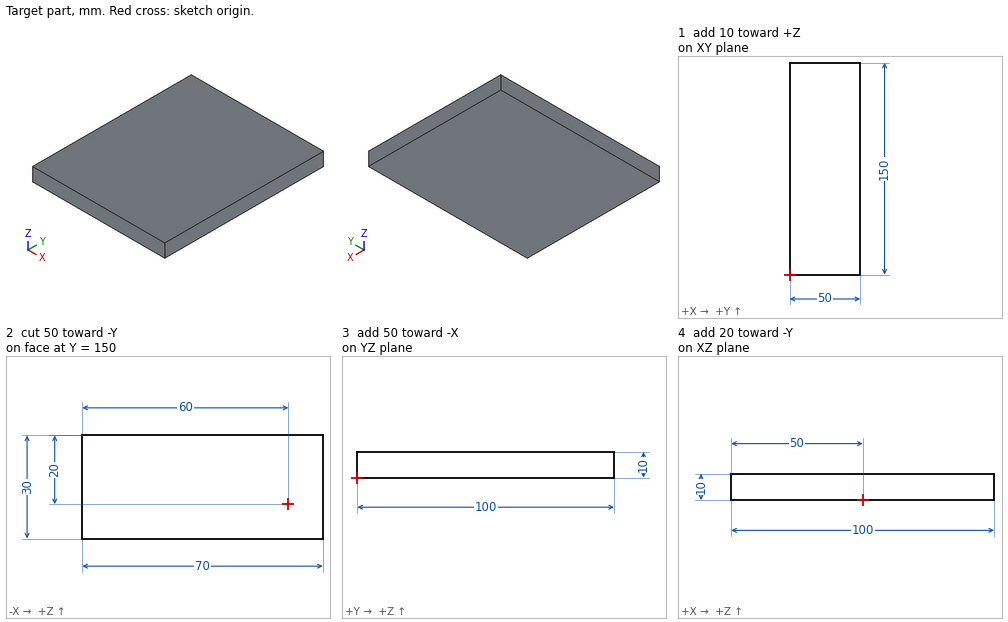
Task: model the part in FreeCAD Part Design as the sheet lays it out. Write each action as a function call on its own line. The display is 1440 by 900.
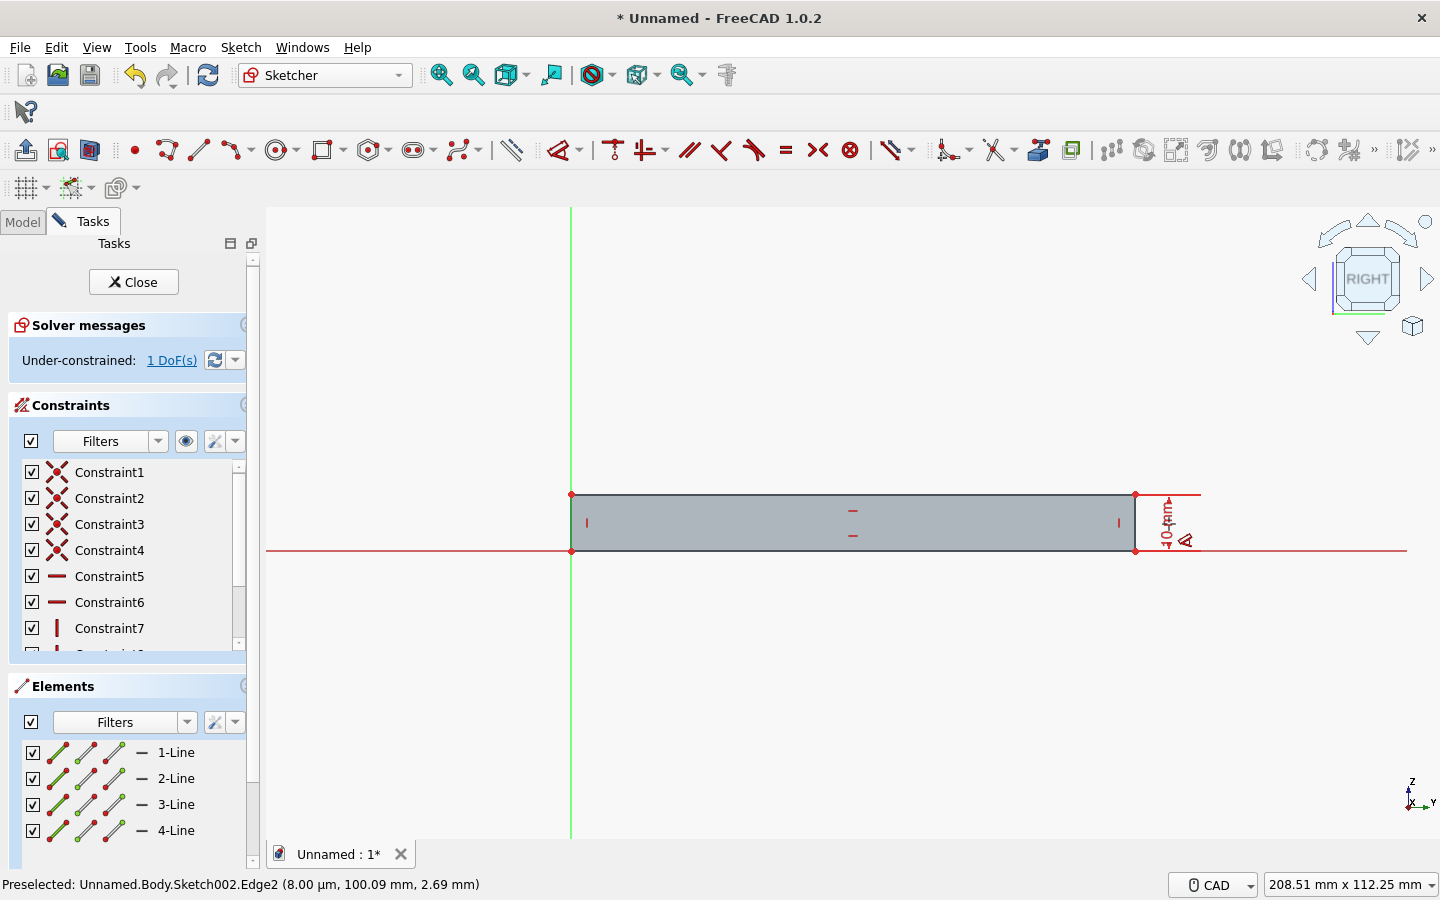
click(741, 551)
click(853, 585)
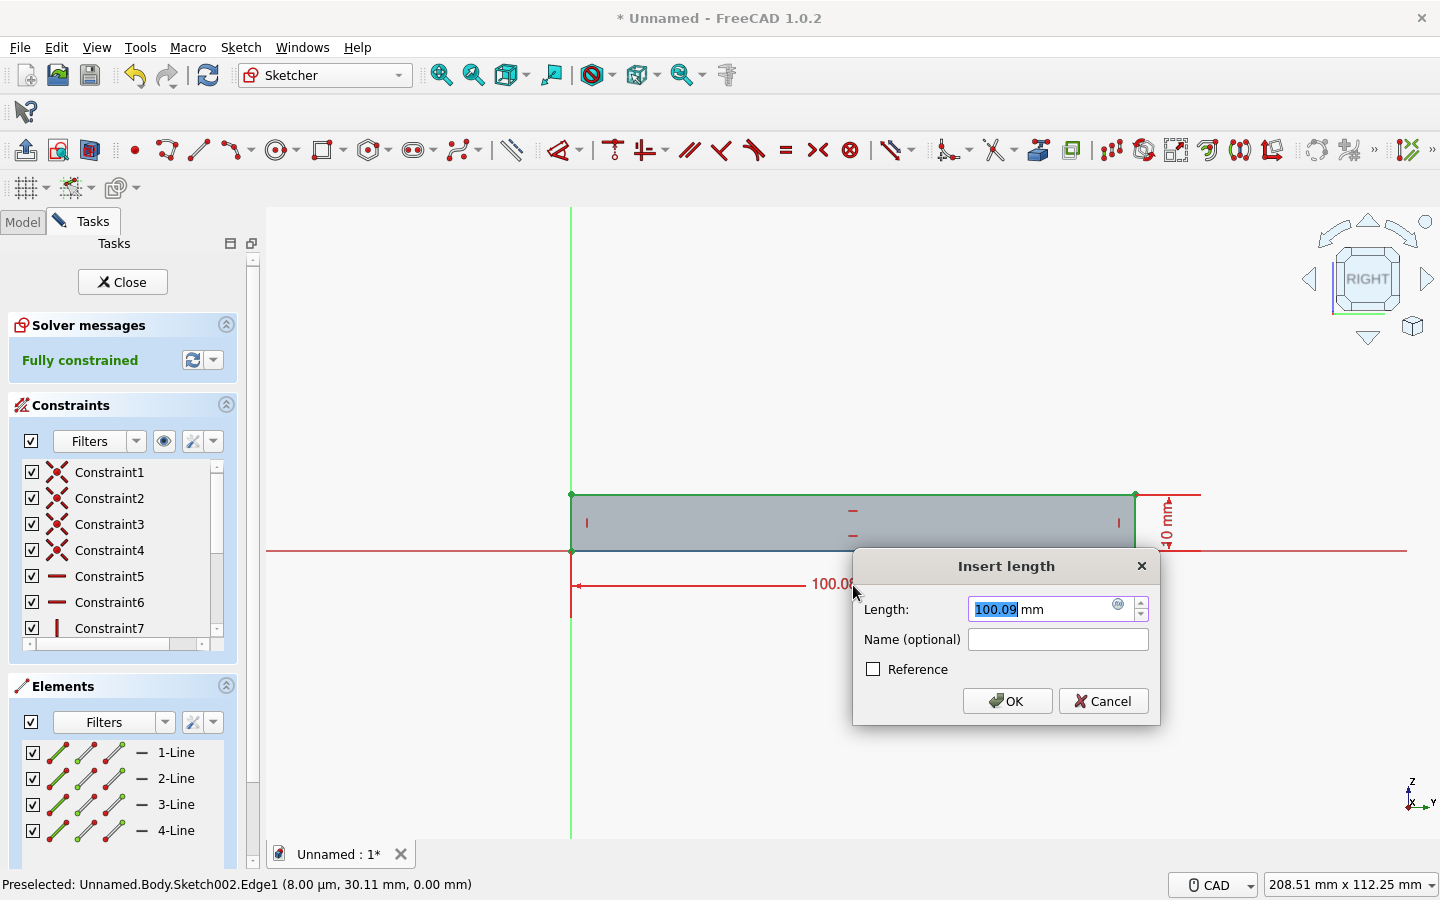
text(100)
key(Return)
key(Escape)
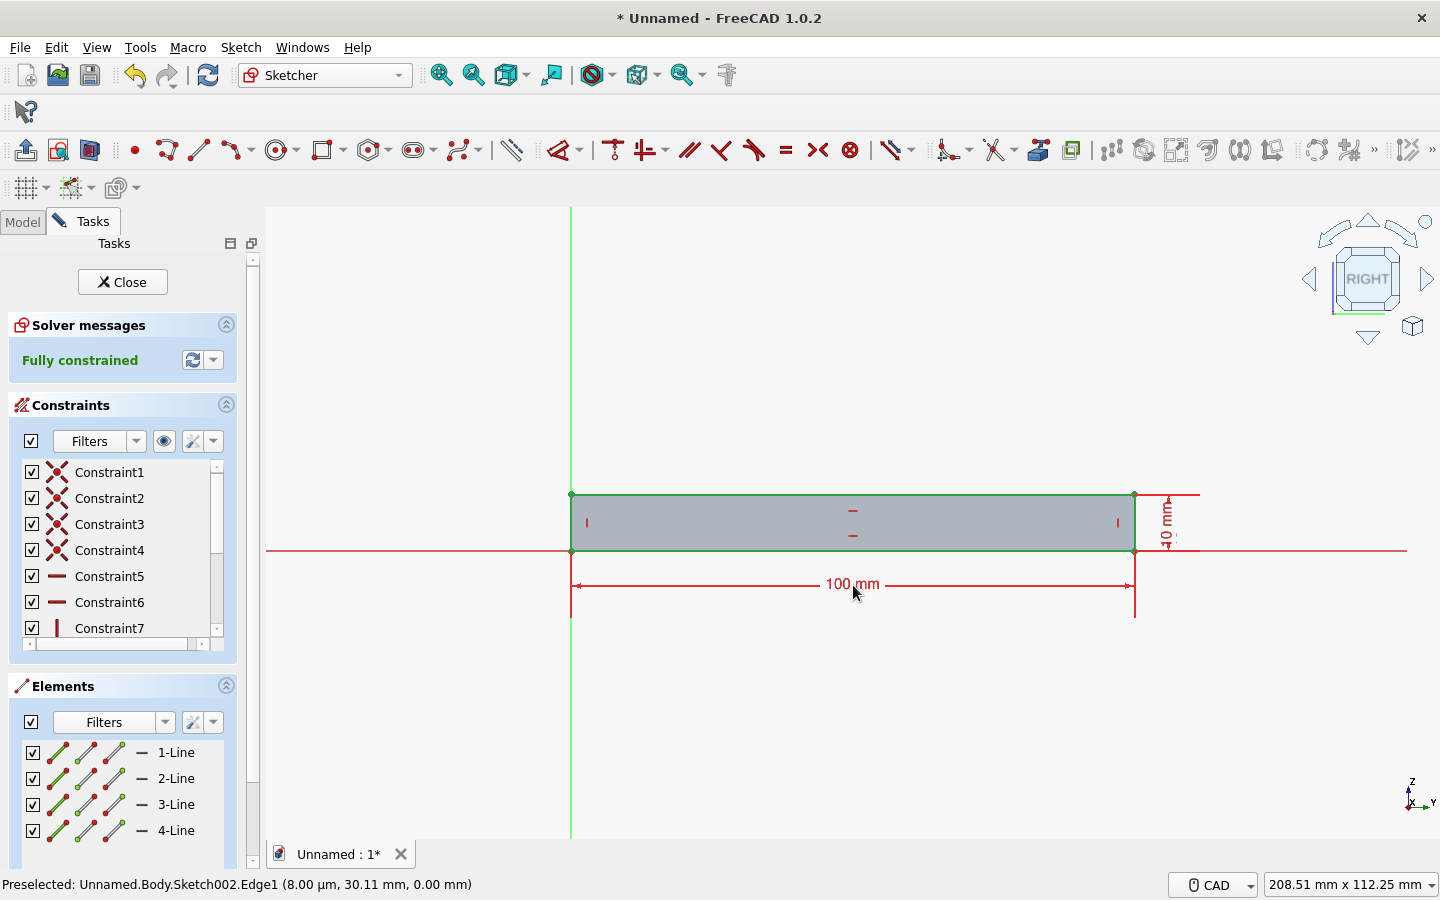
click(123, 282)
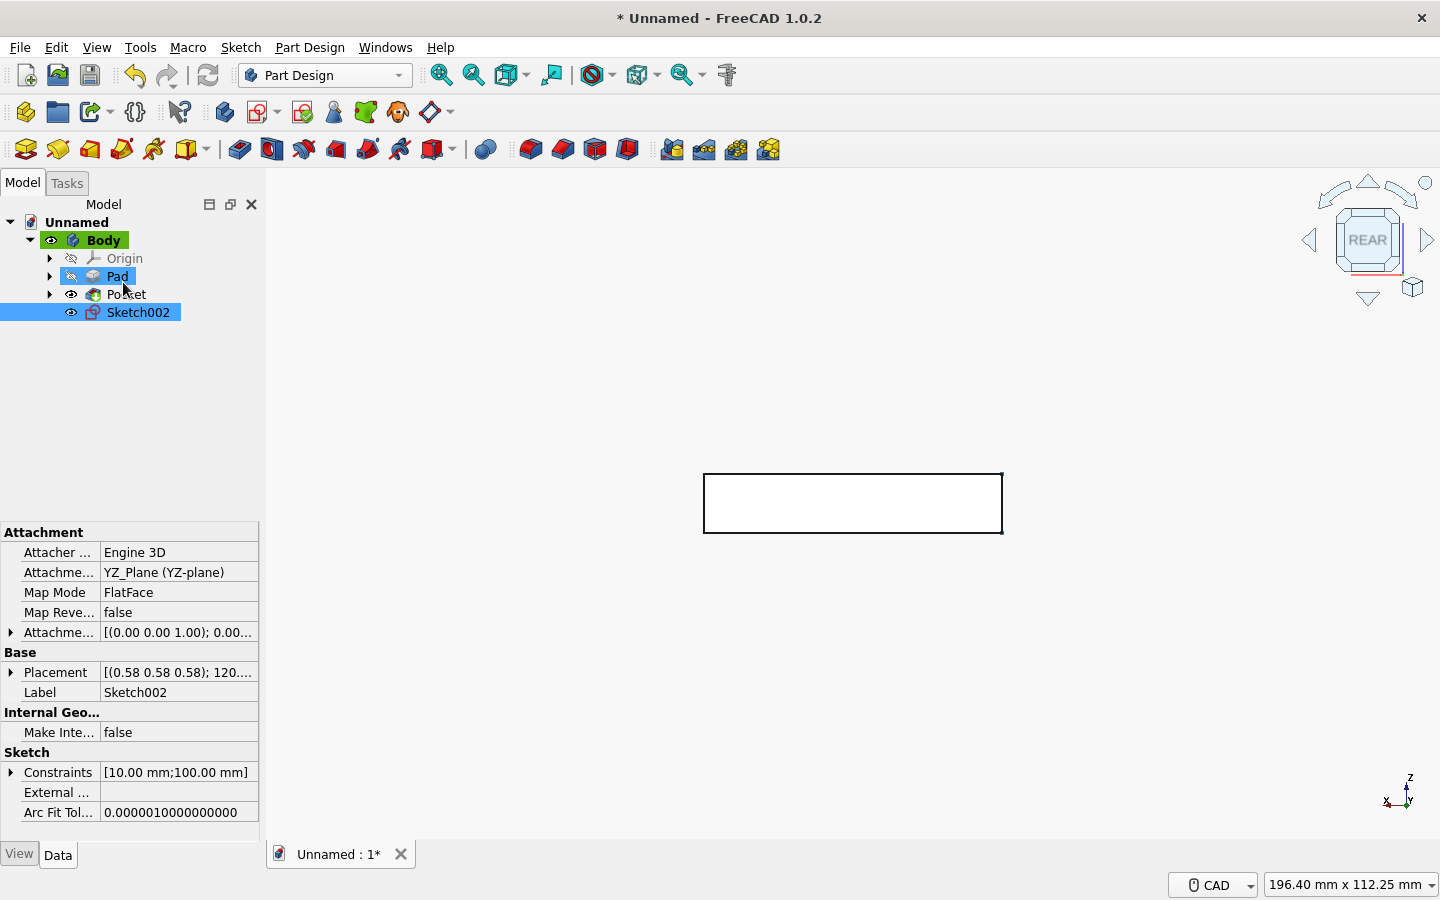
click(26, 150)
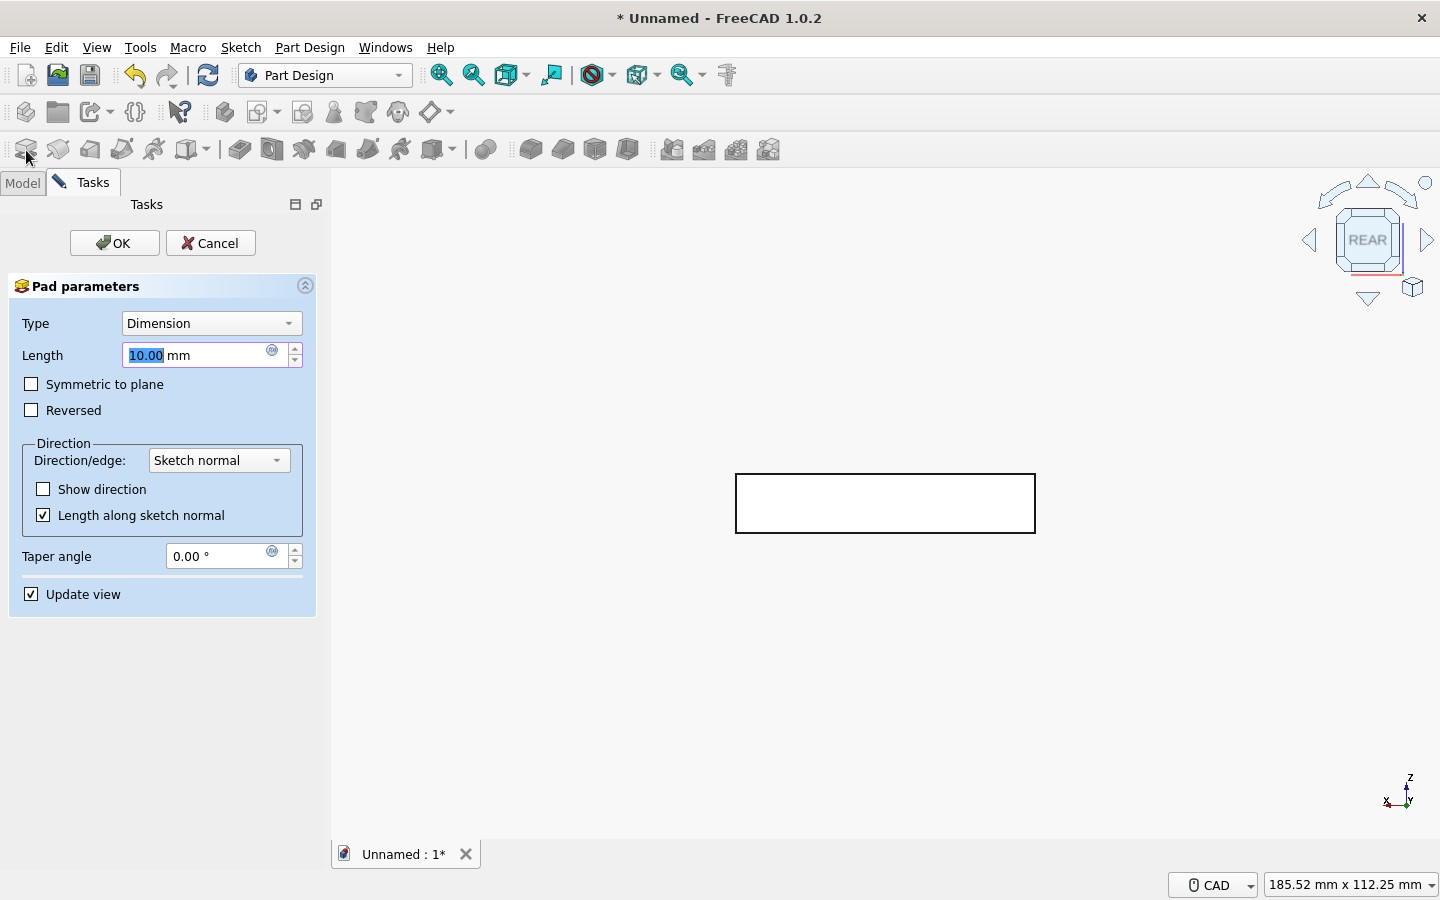
text(50)
key(Tab)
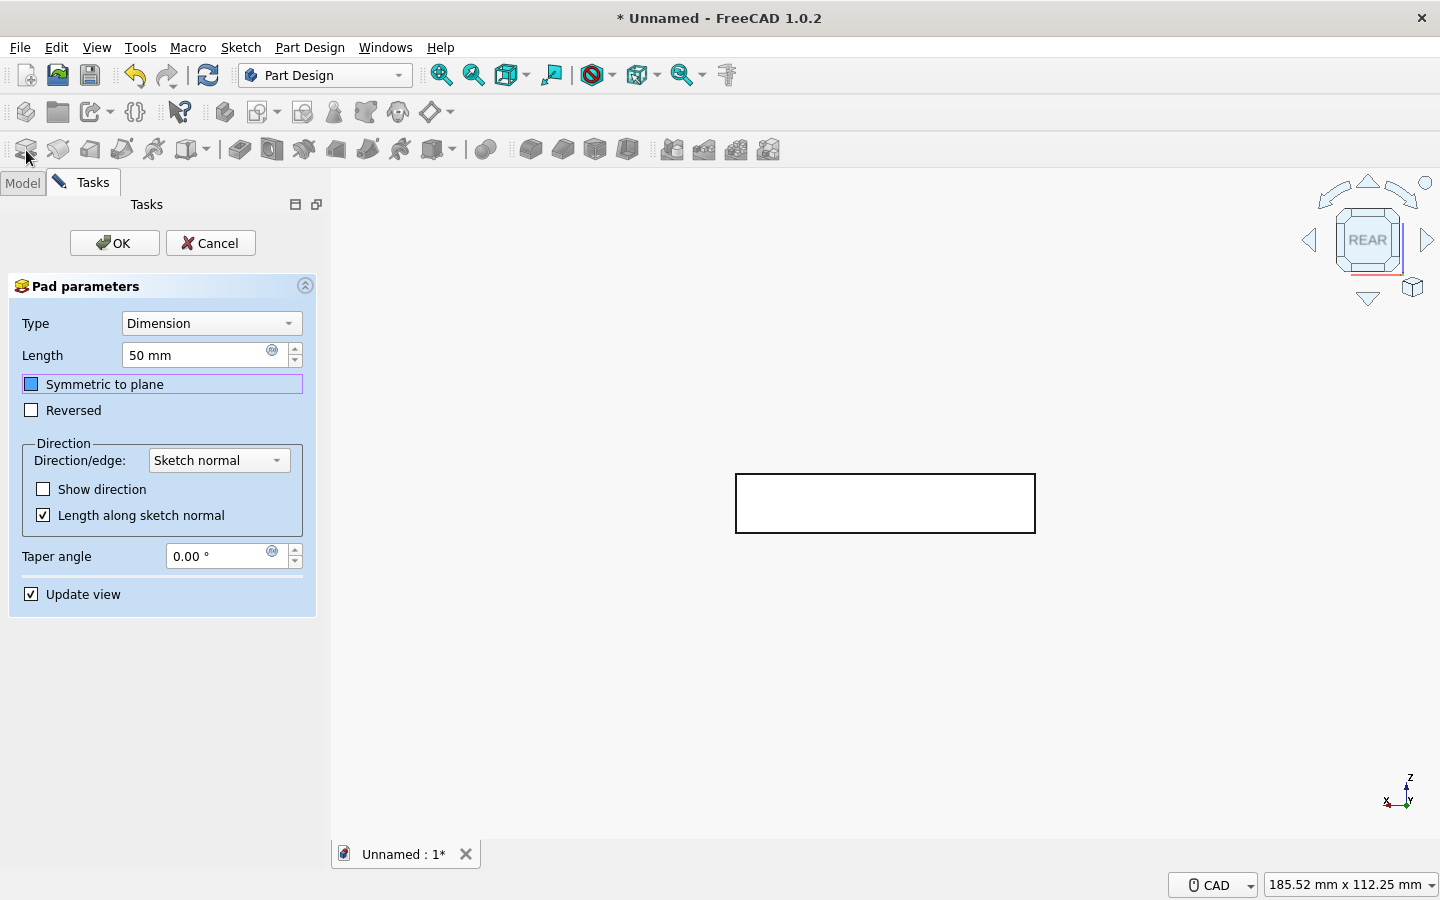
click(30, 410)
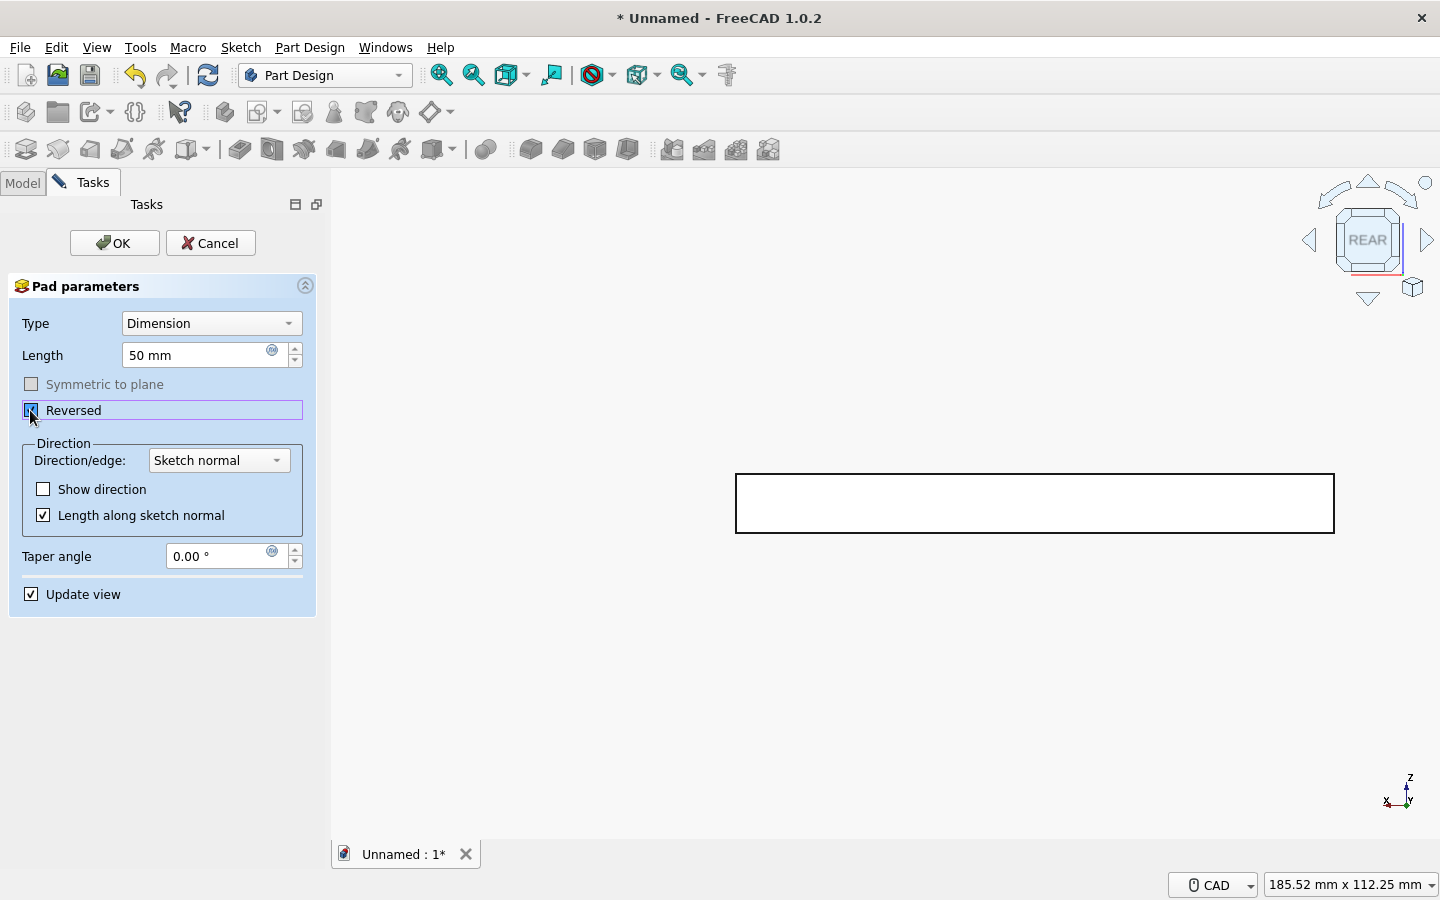
click(115, 243)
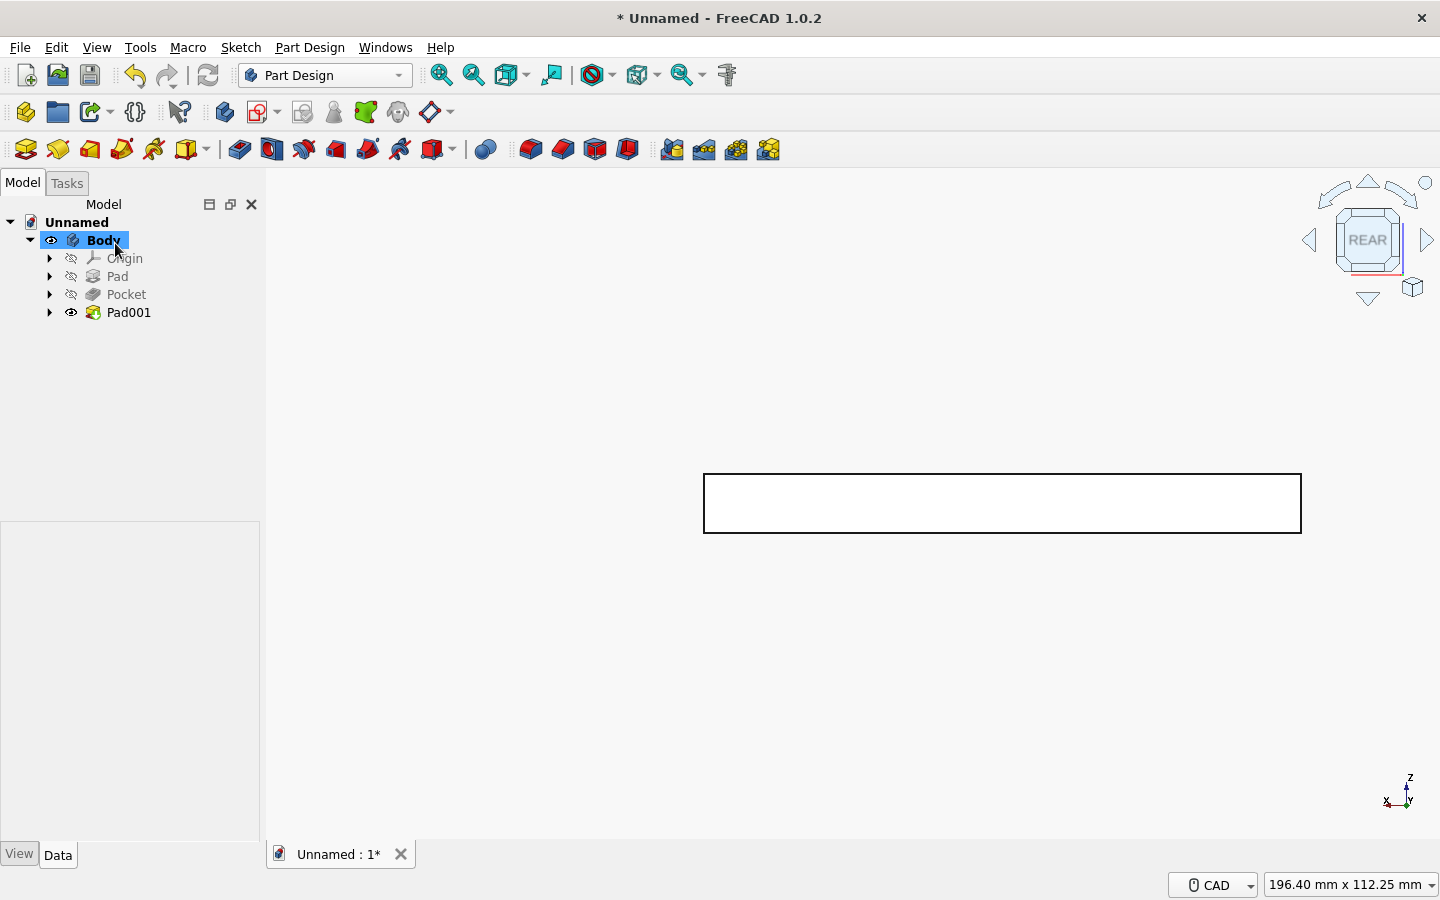
click(258, 112)